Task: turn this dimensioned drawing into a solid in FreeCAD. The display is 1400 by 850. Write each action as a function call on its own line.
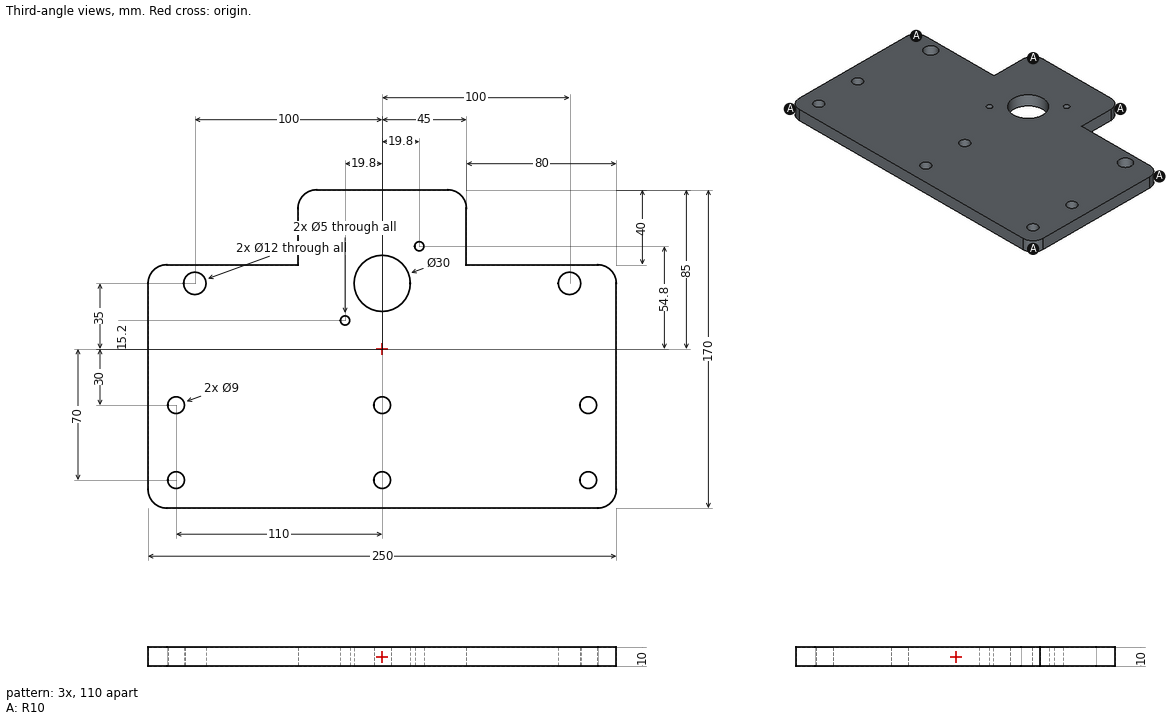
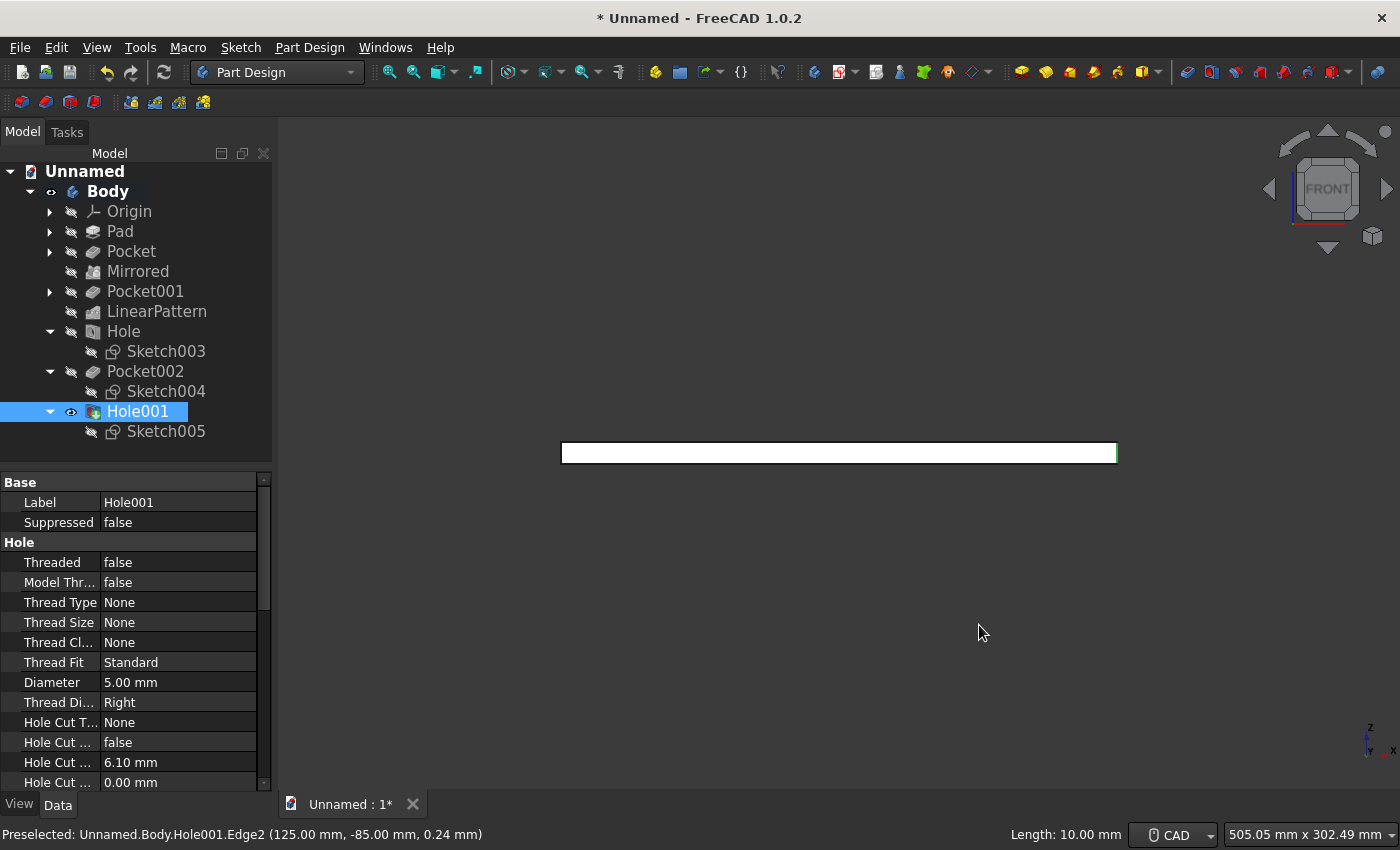
click(561, 452, ctrl)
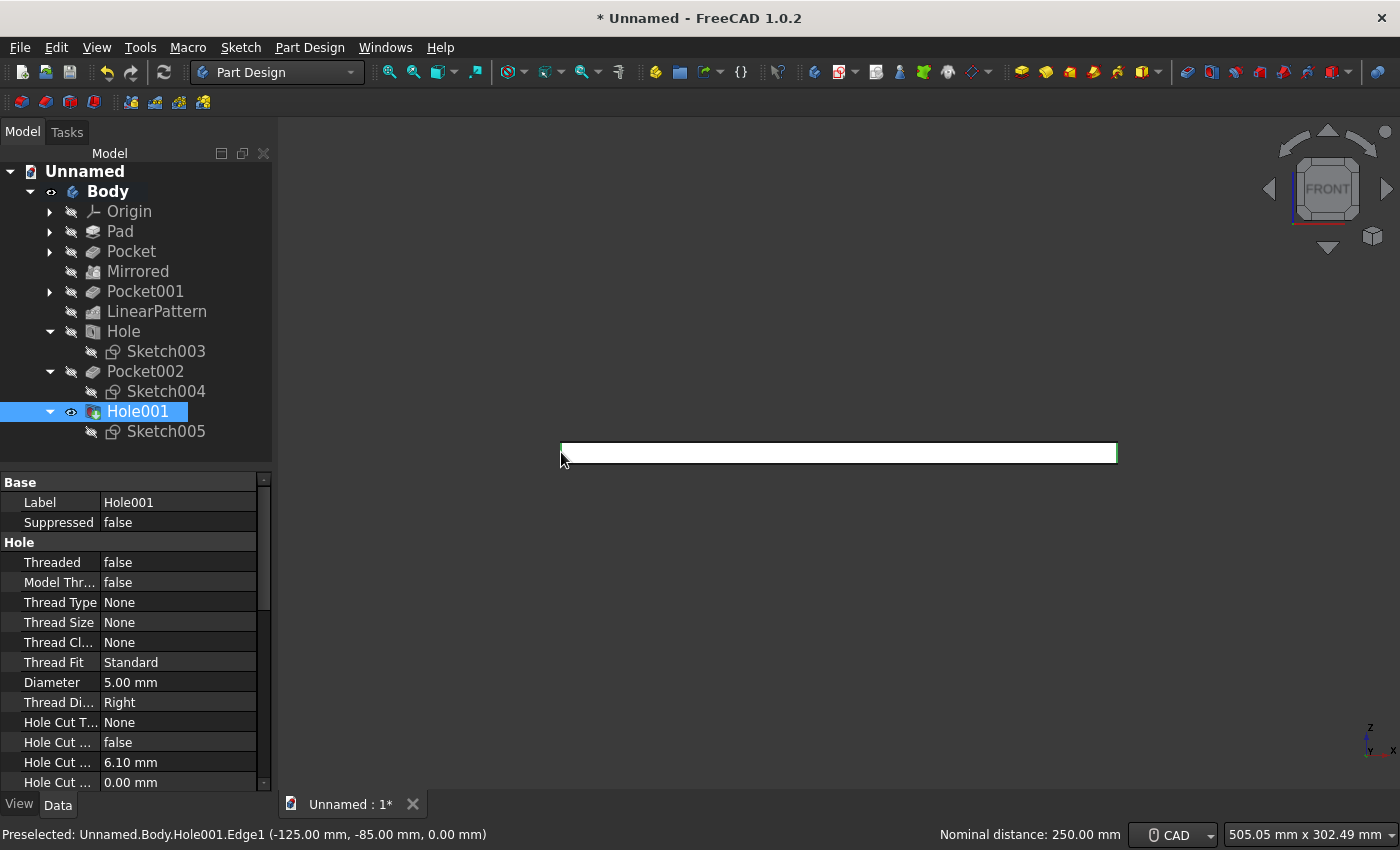
key(3)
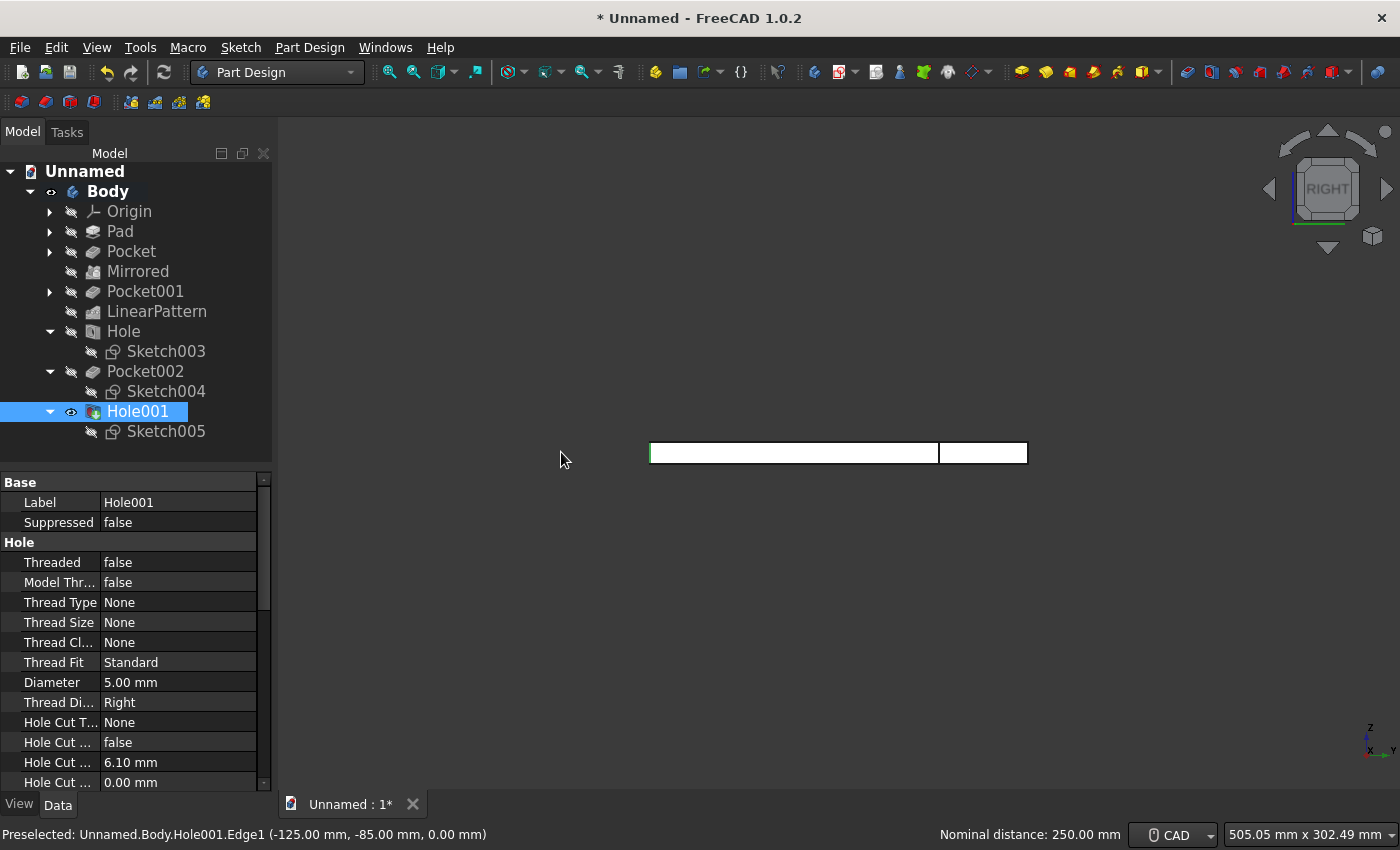
click(390, 72)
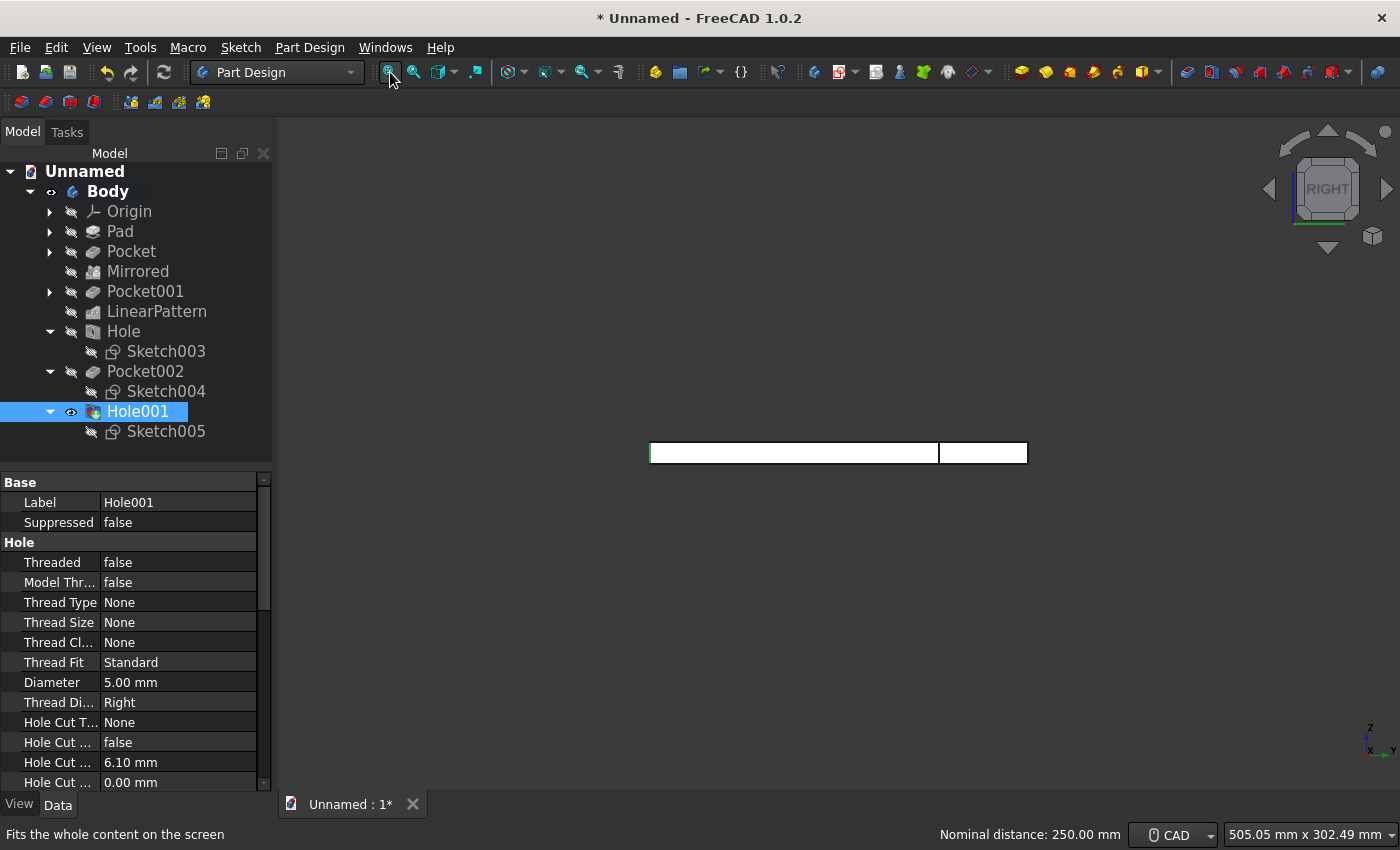
click(1028, 452, ctrl)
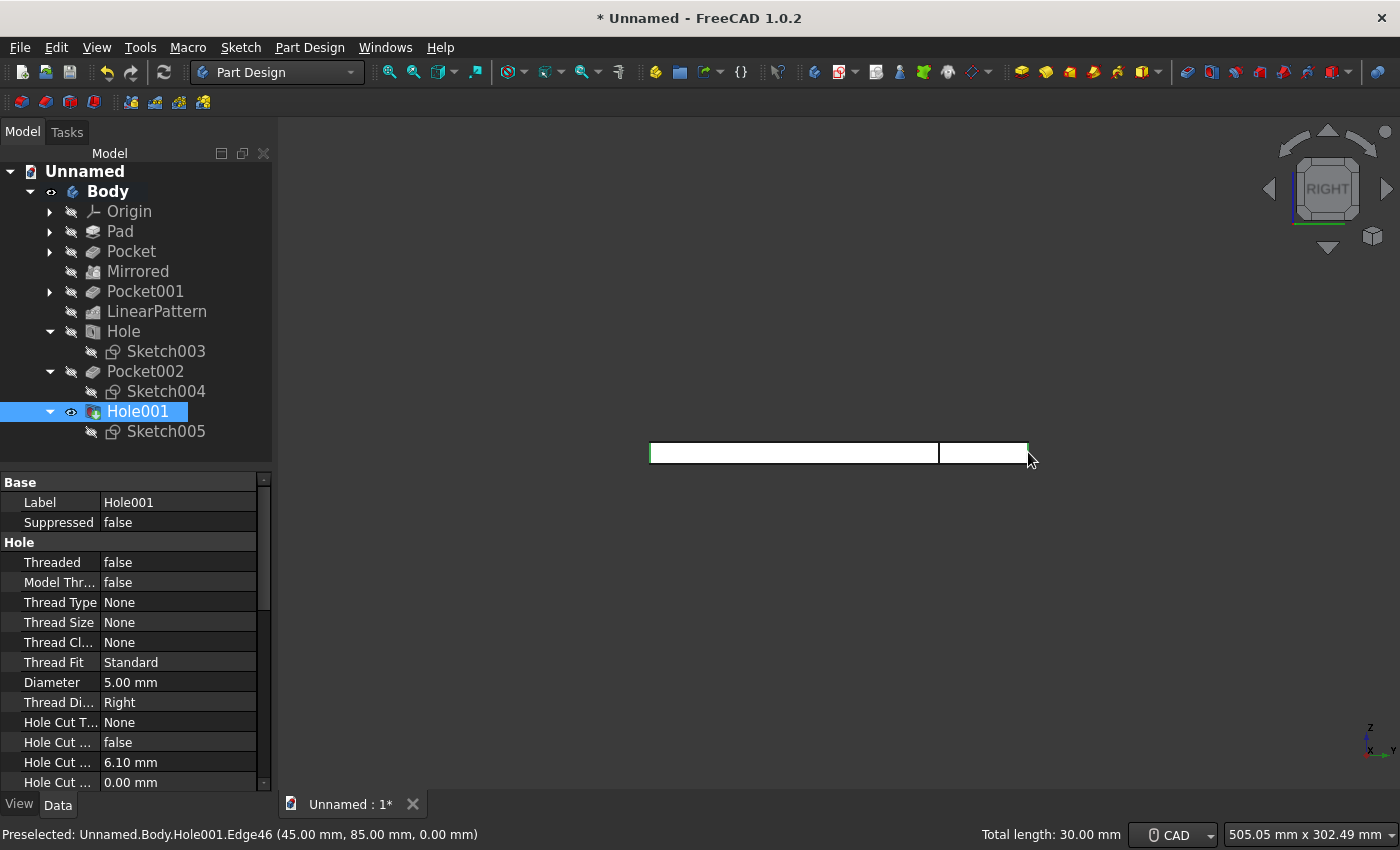
click(939, 452, ctrl)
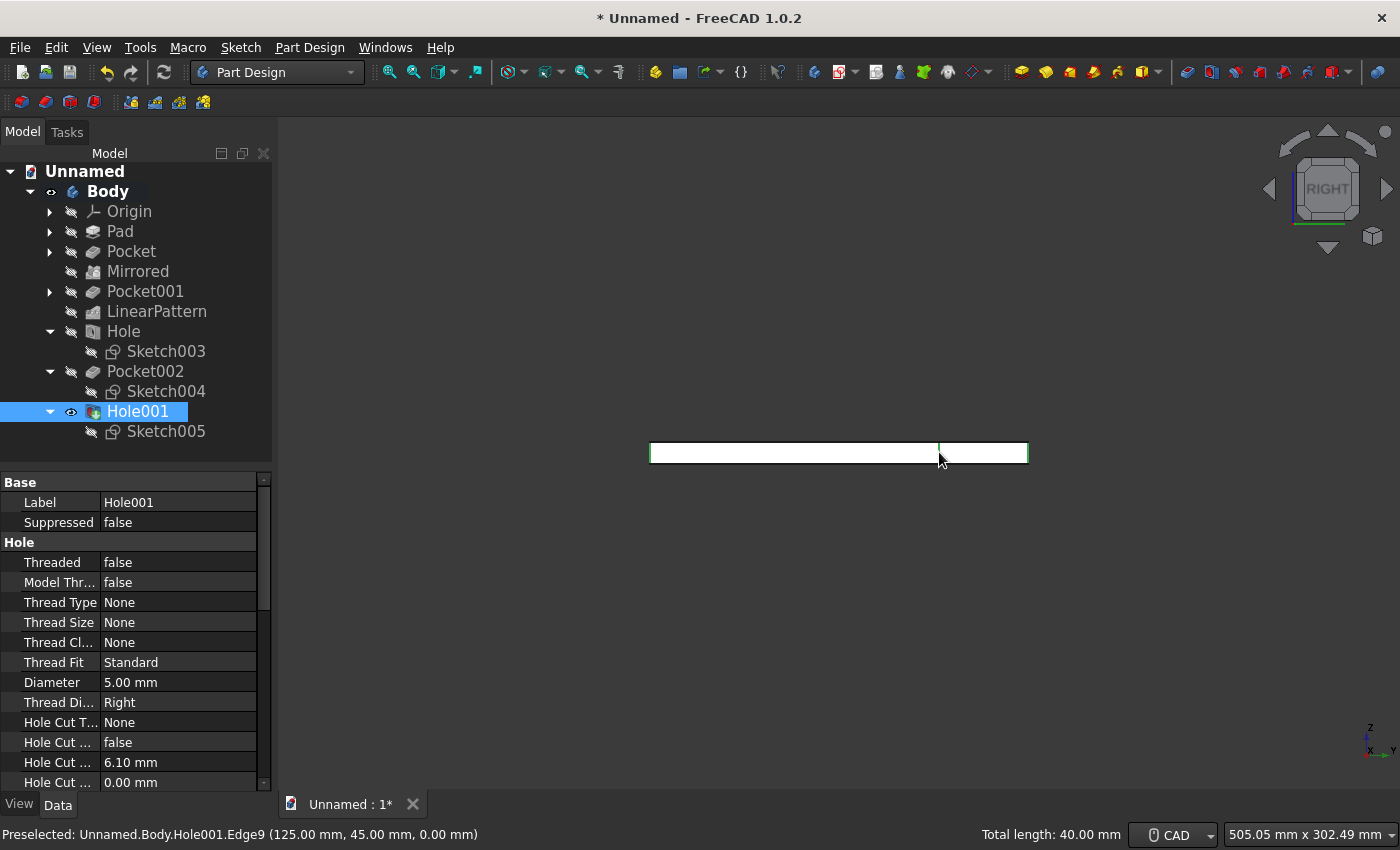
key(5)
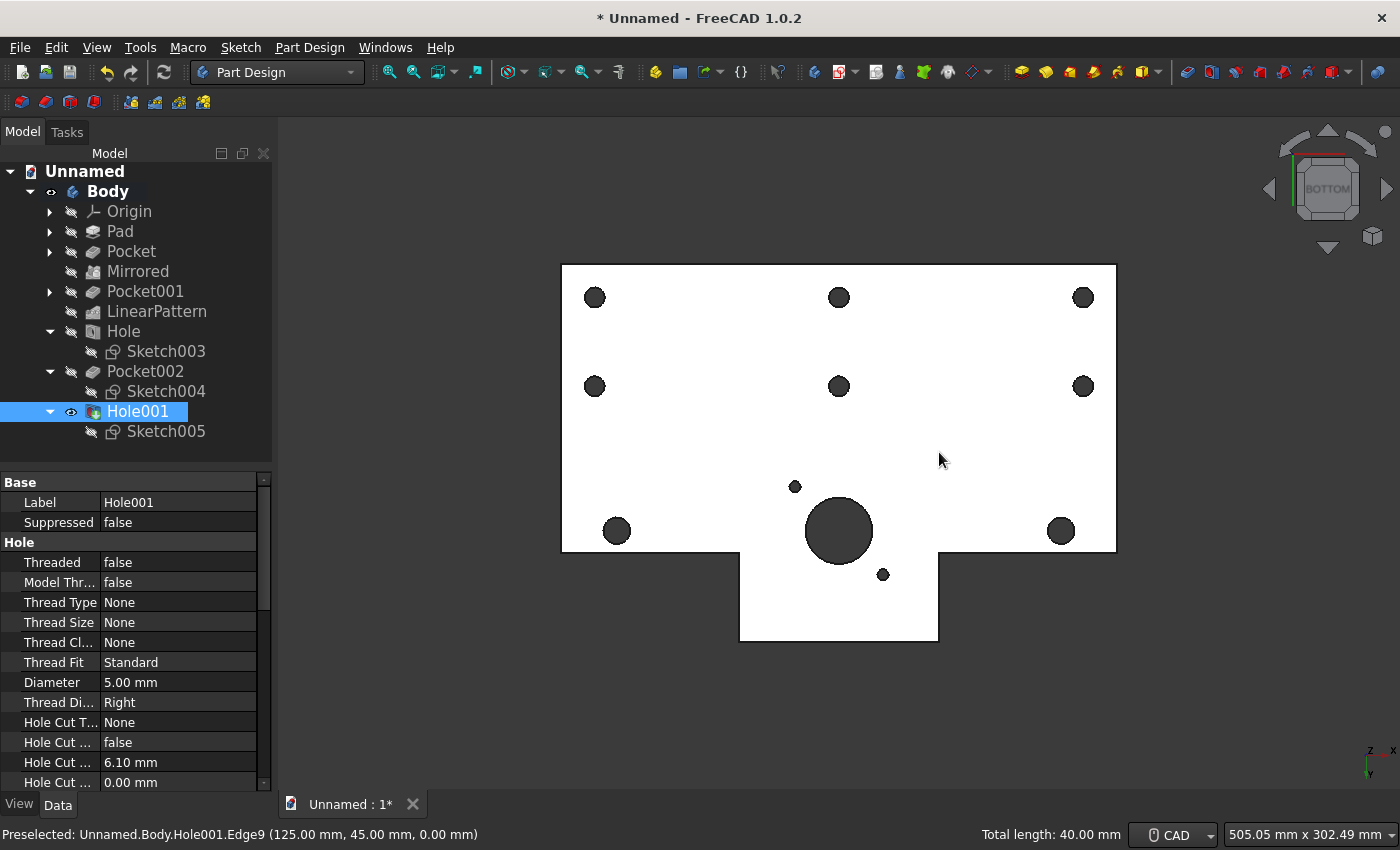
key(4)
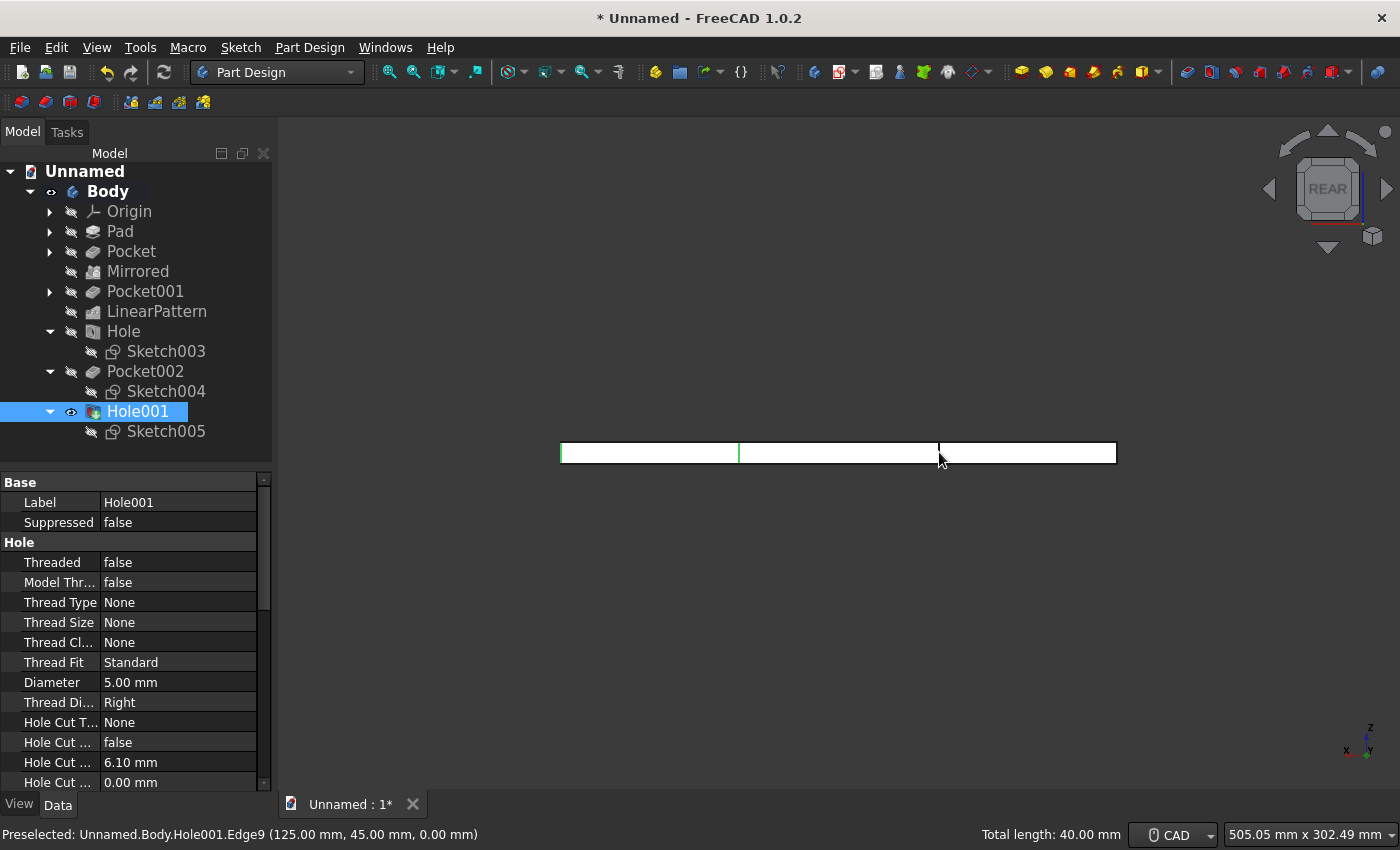
click(939, 452, ctrl)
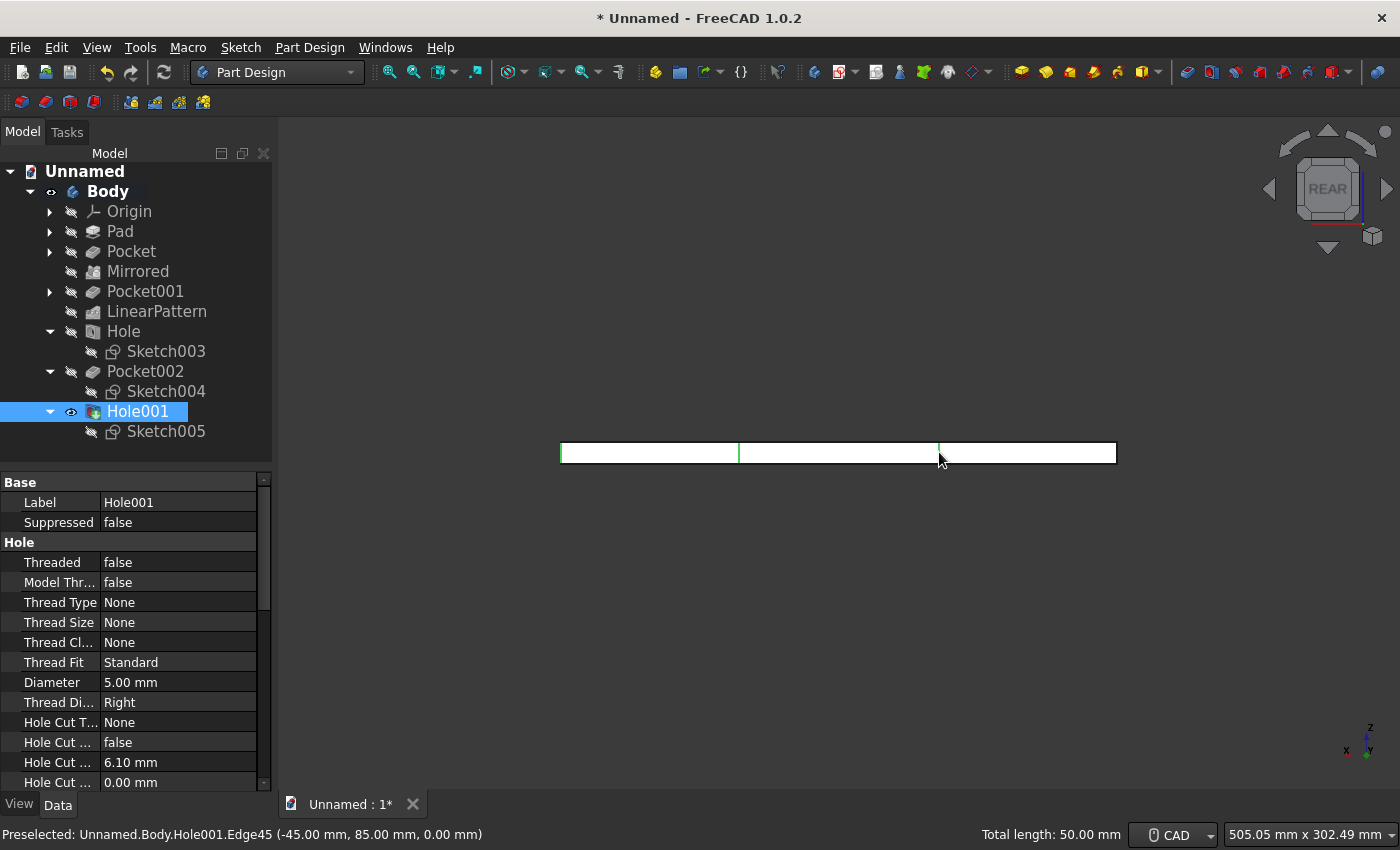
click(1117, 452, ctrl)